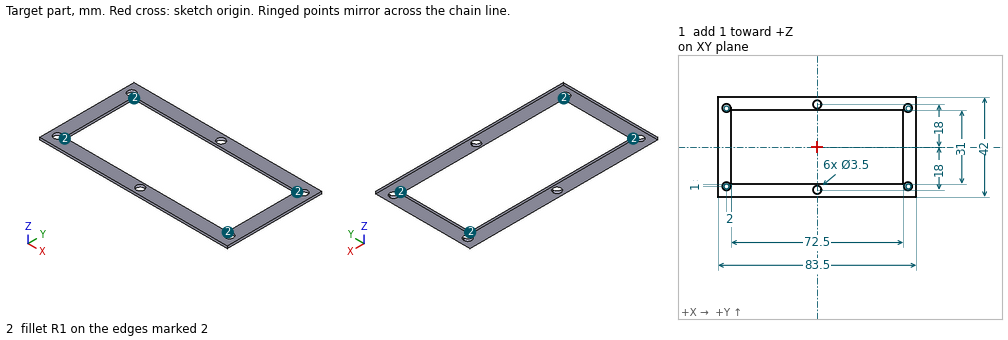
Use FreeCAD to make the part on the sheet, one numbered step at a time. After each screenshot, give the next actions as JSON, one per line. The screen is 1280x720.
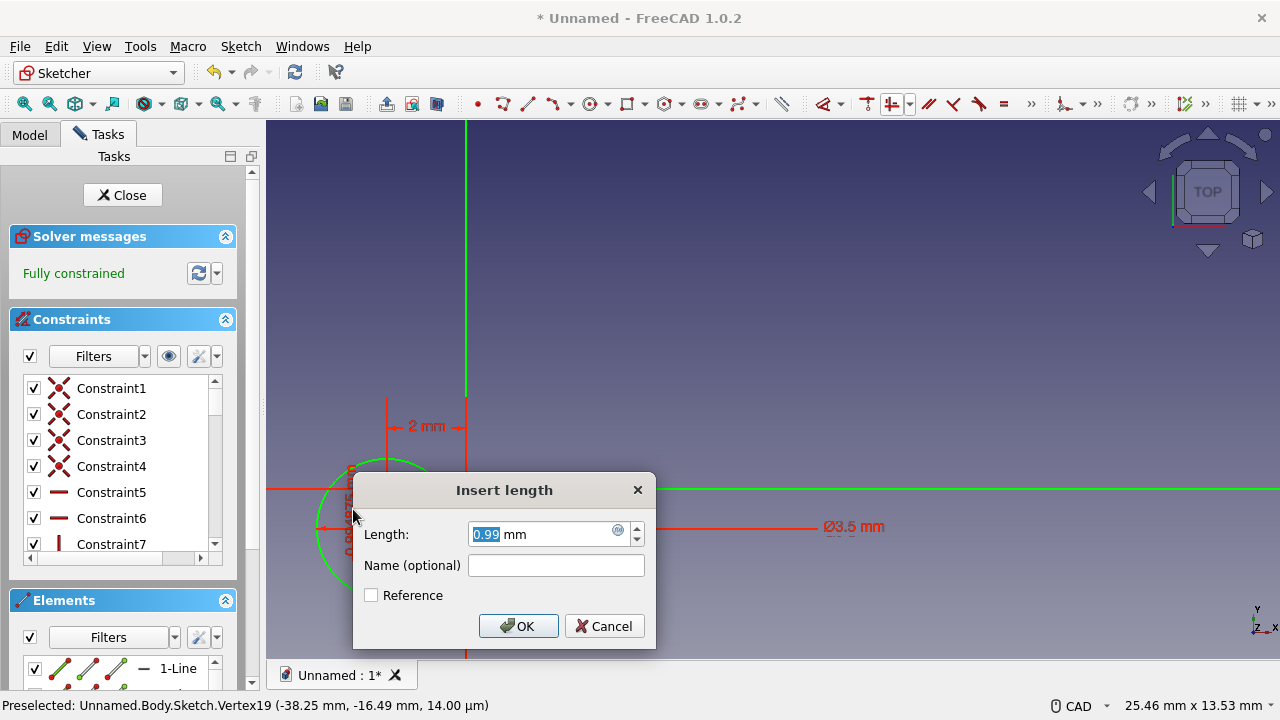
{"action": "type", "text": "1"}
{"action": "key", "text": "Return"}
{"action": "key", "text": "Escape"}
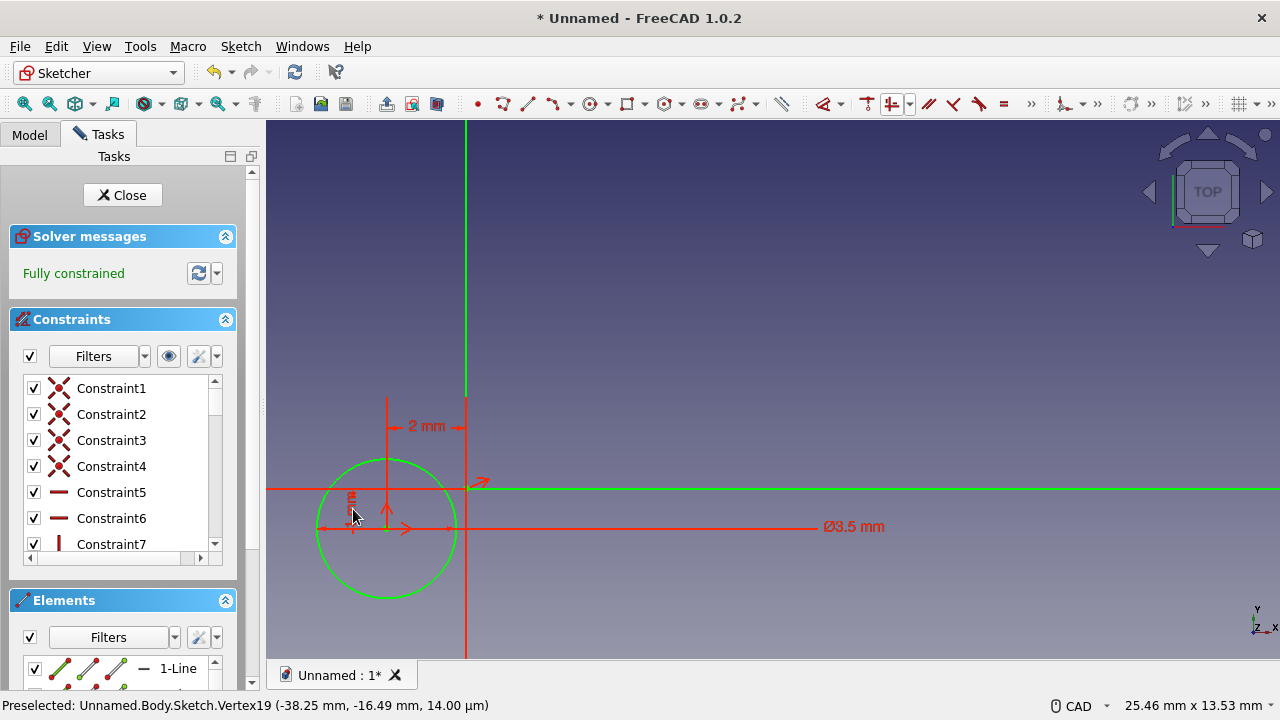
{"action": "left_click", "coordinate": [123, 195]}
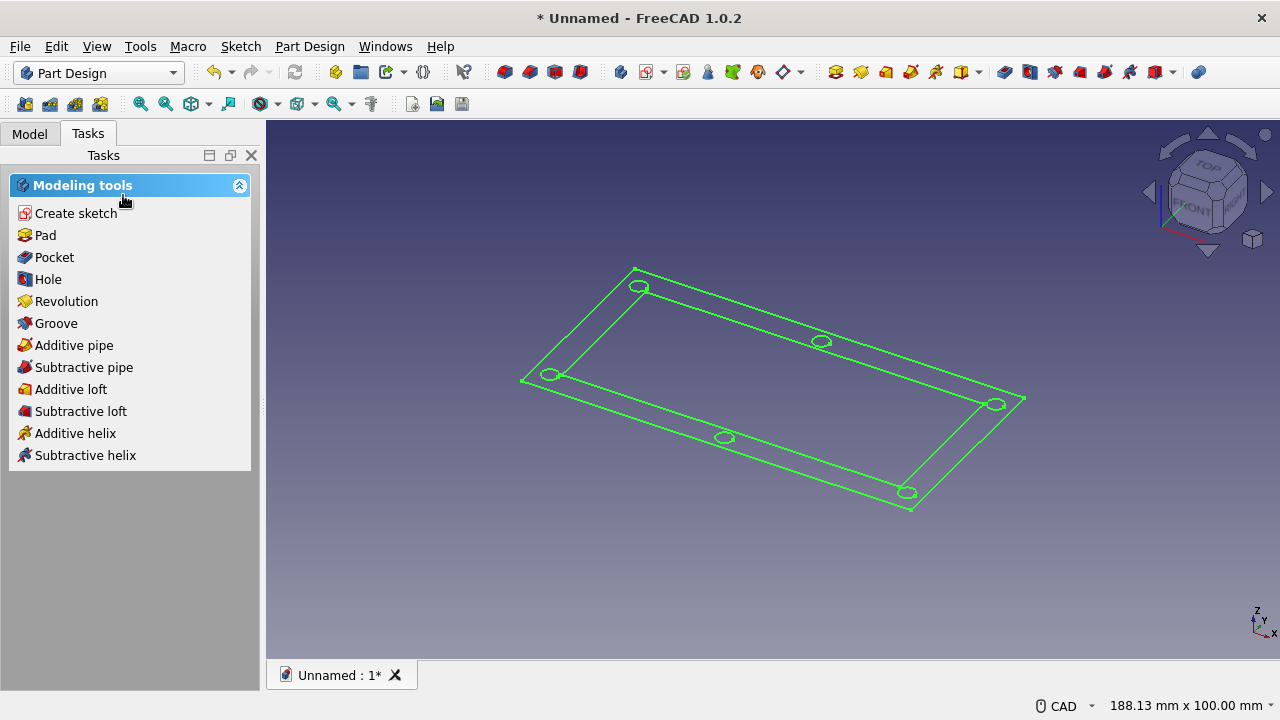
{"action": "left_click", "coordinate": [836, 72]}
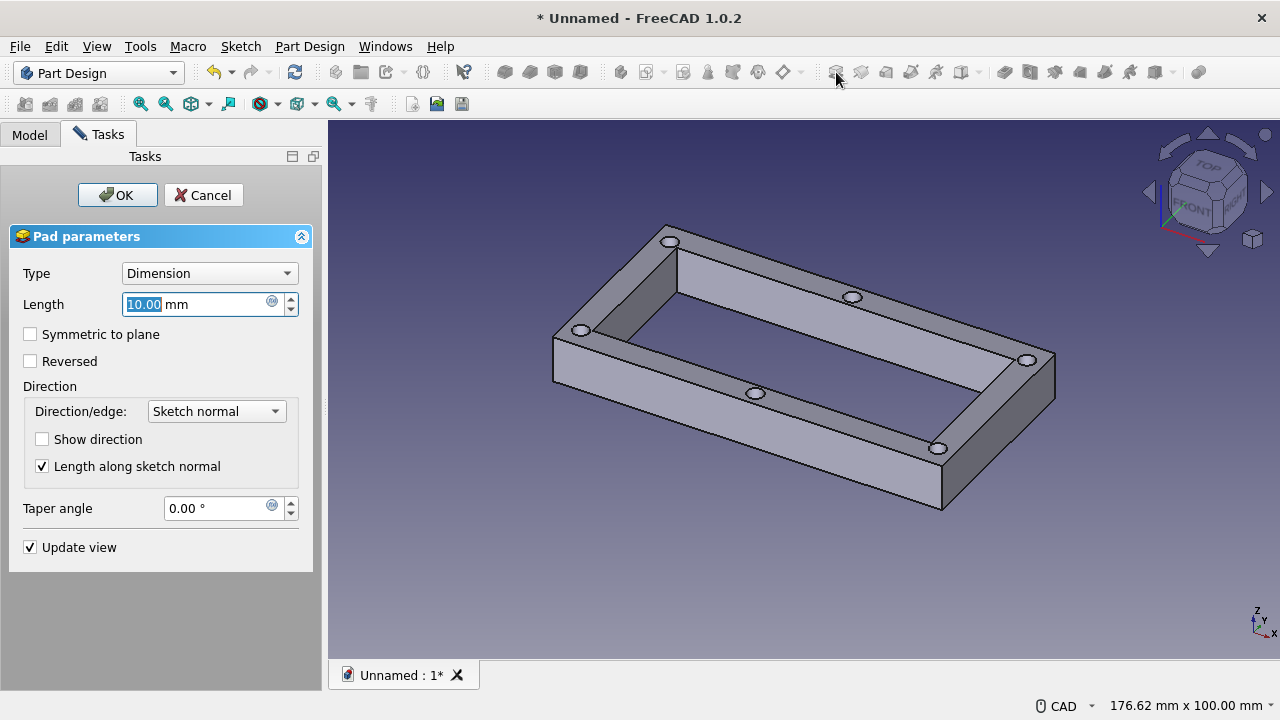
{"action": "type", "text": "1"}
{"action": "key", "text": "Tab"}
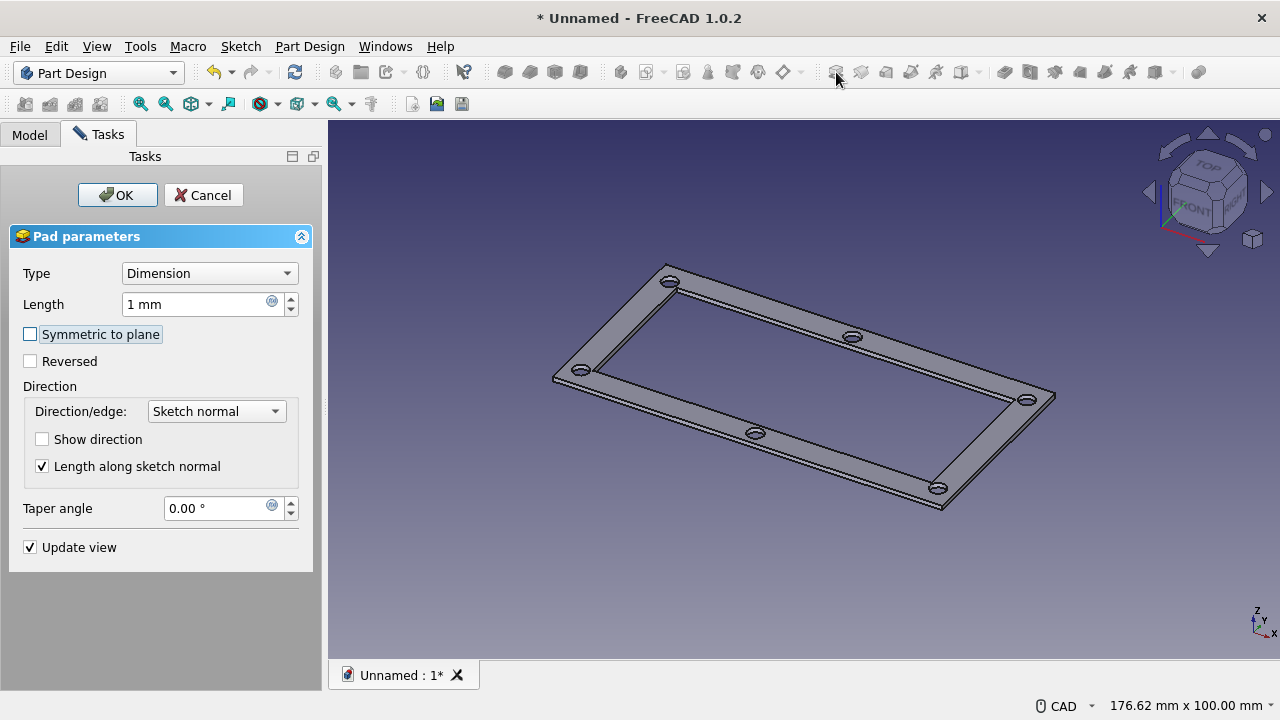
{"action": "left_click", "coordinate": [118, 195]}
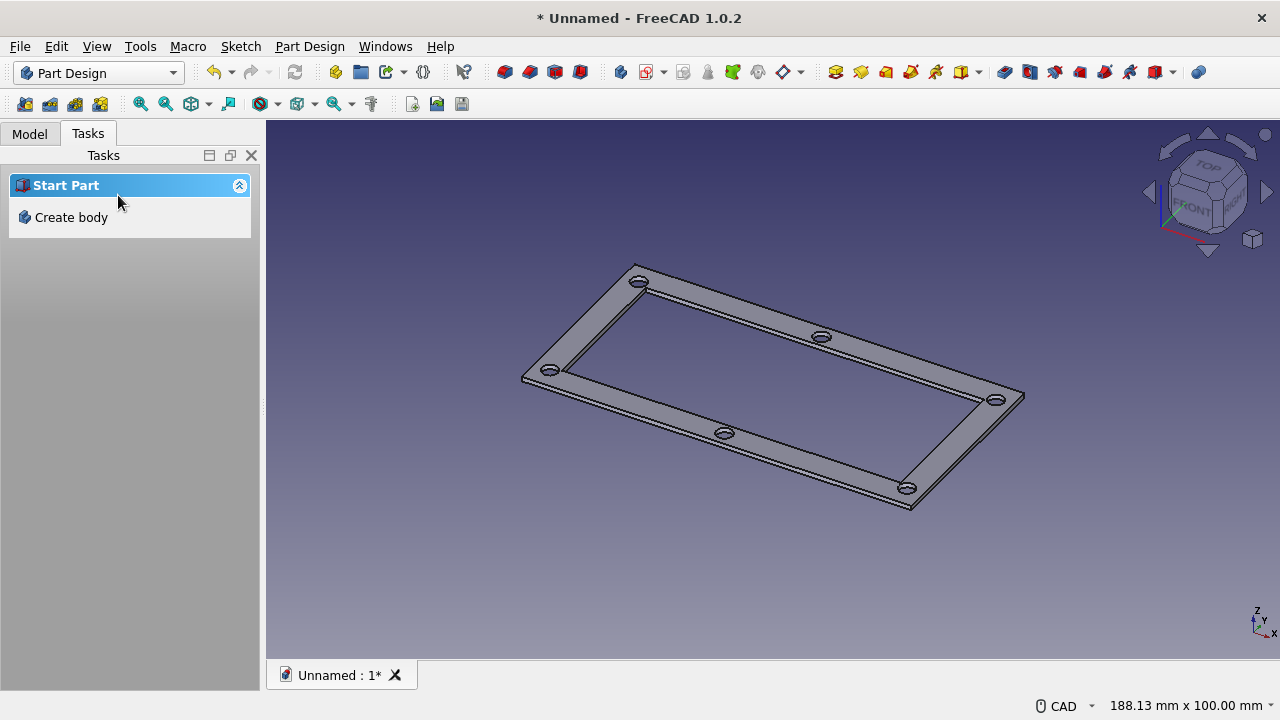
{"action": "scroll", "coordinate": [646, 289], "scroll_direction": "up", "scroll_amount": 11}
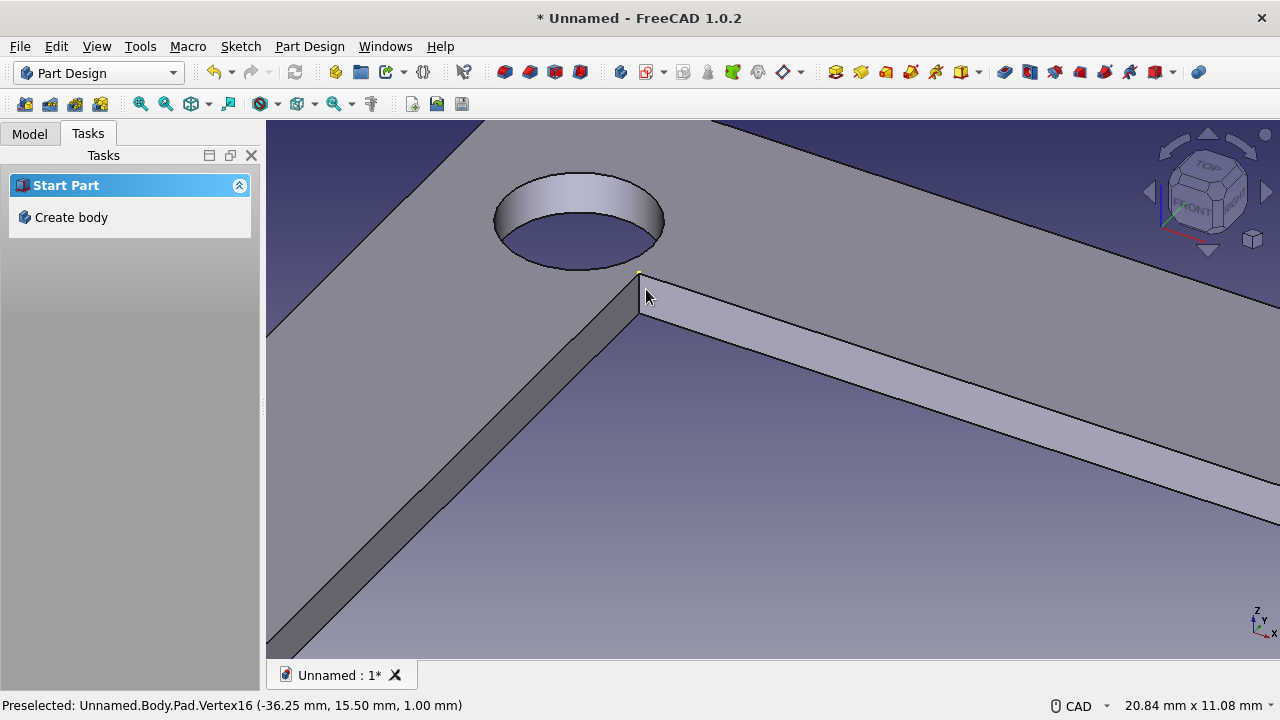
{"action": "key", "text": "v f"}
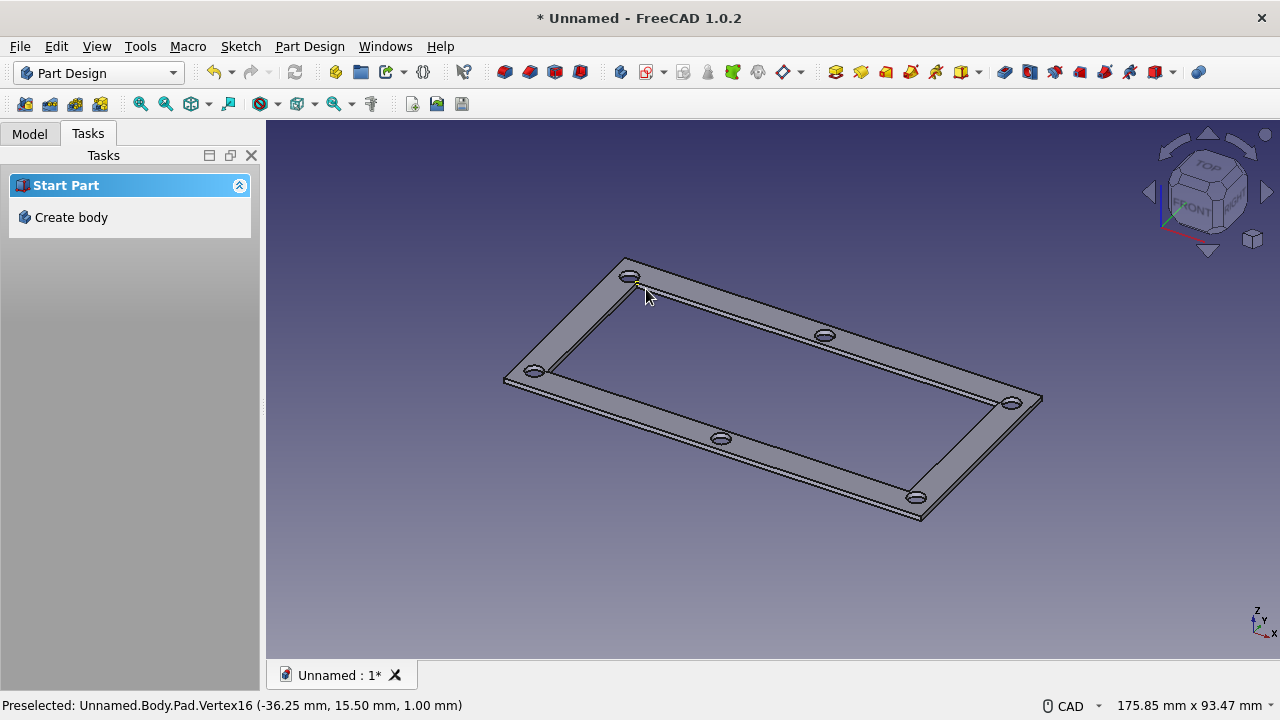
{"action": "key", "text": "0"}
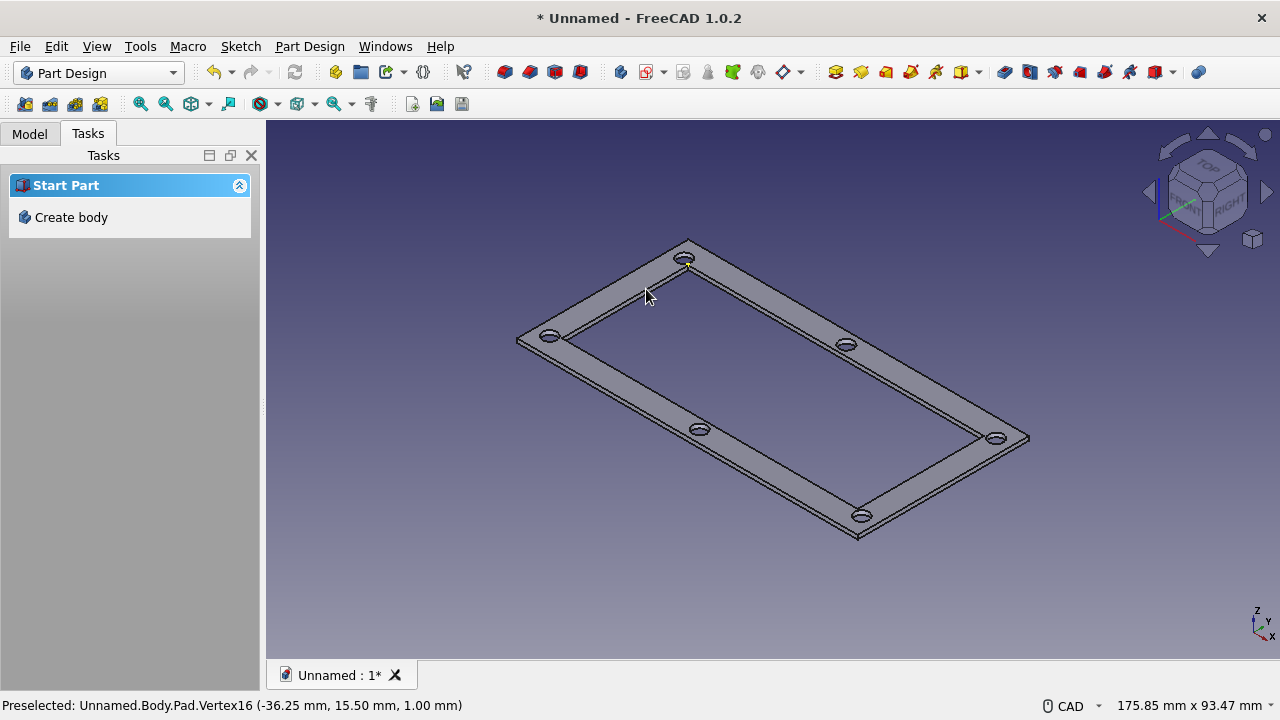
{"action": "scroll", "coordinate": [688, 267], "scroll_direction": "up", "scroll_amount": 10}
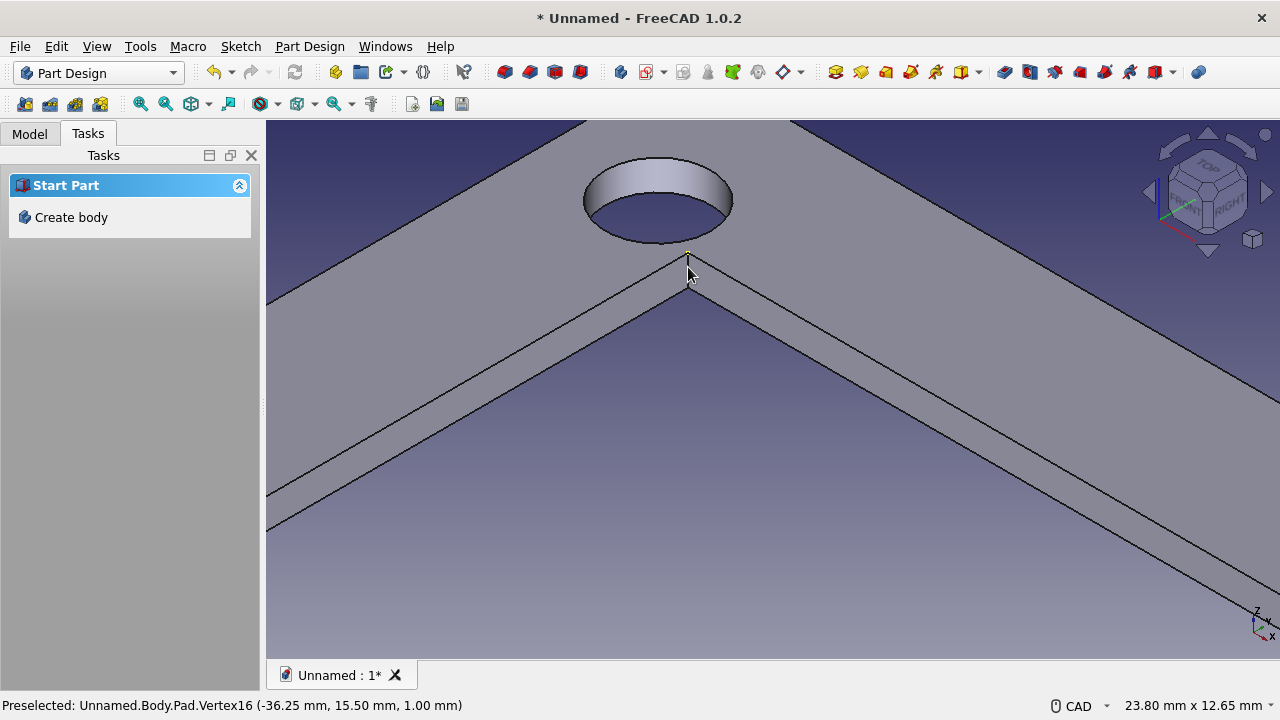
{"action": "key", "text": "v f"}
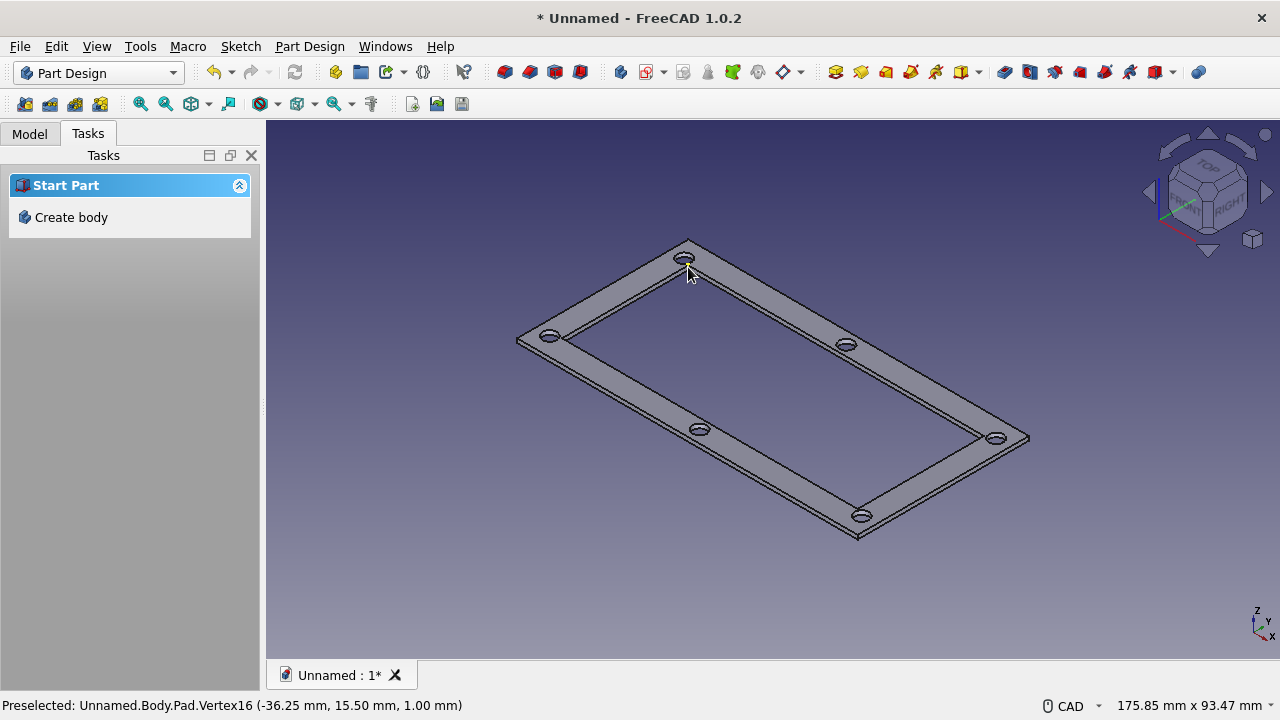
{"action": "key", "text": "2"}